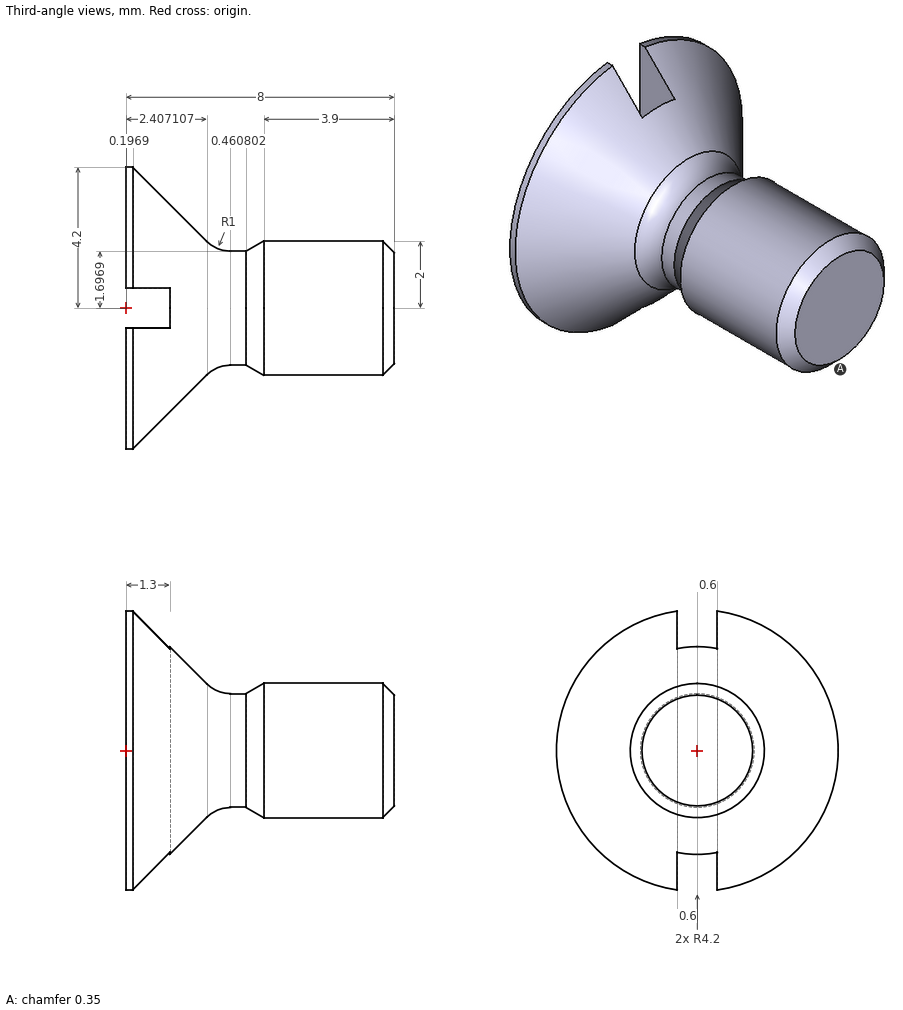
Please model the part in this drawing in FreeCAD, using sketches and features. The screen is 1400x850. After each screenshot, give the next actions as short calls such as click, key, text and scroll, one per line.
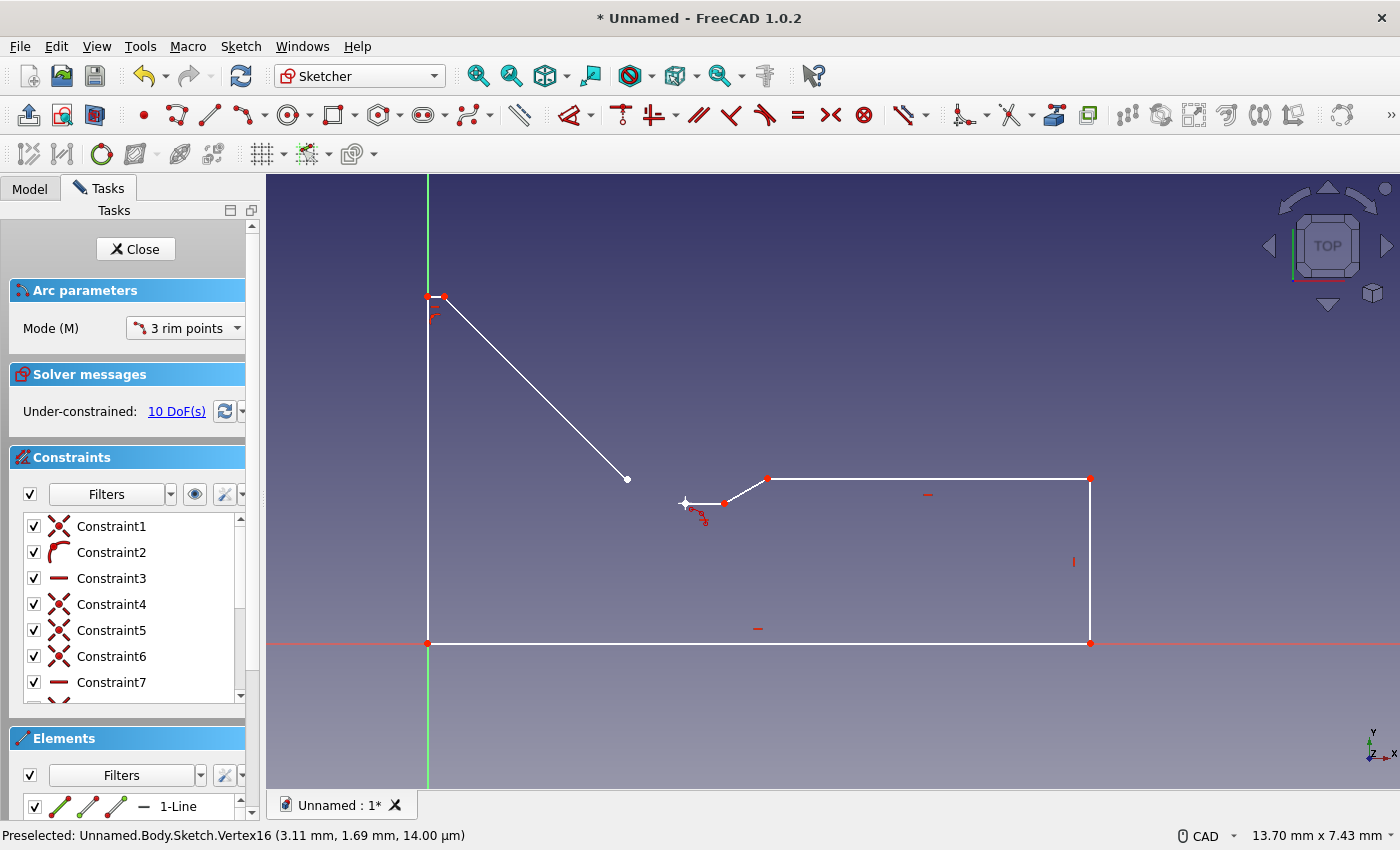
click(685, 504)
click(627, 480)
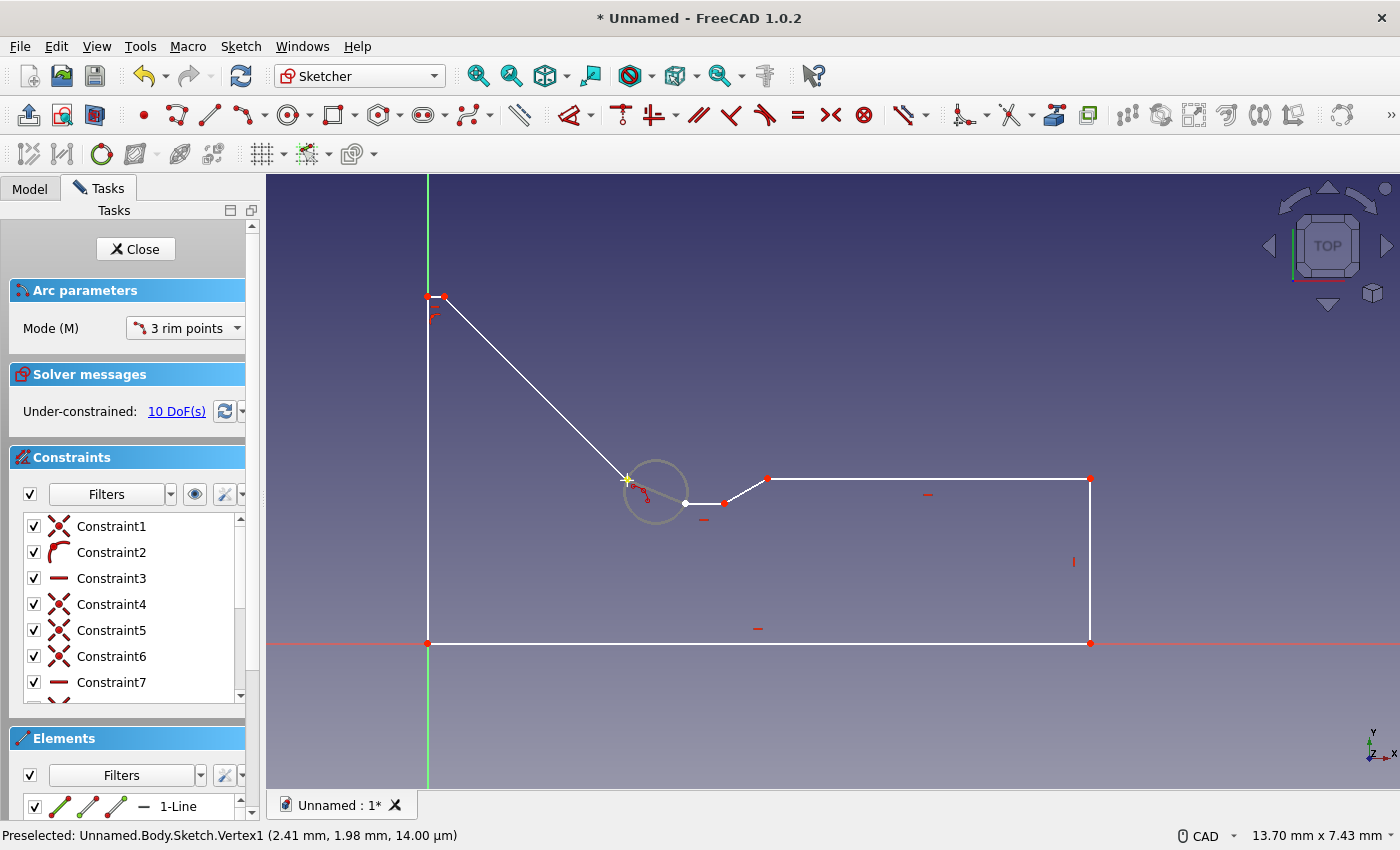
scroll(654, 497, up, 5)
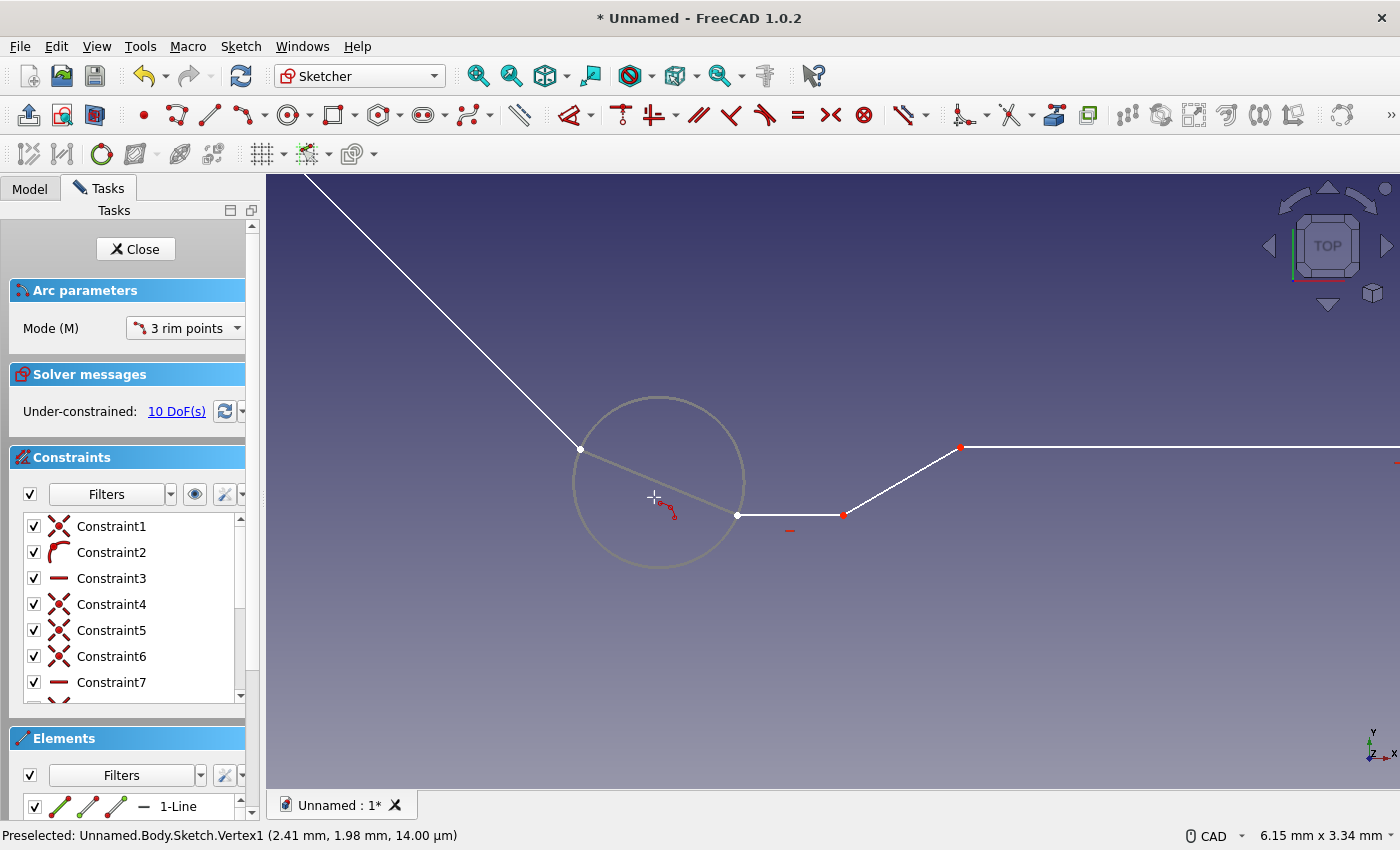
click(653, 496)
key(Escape)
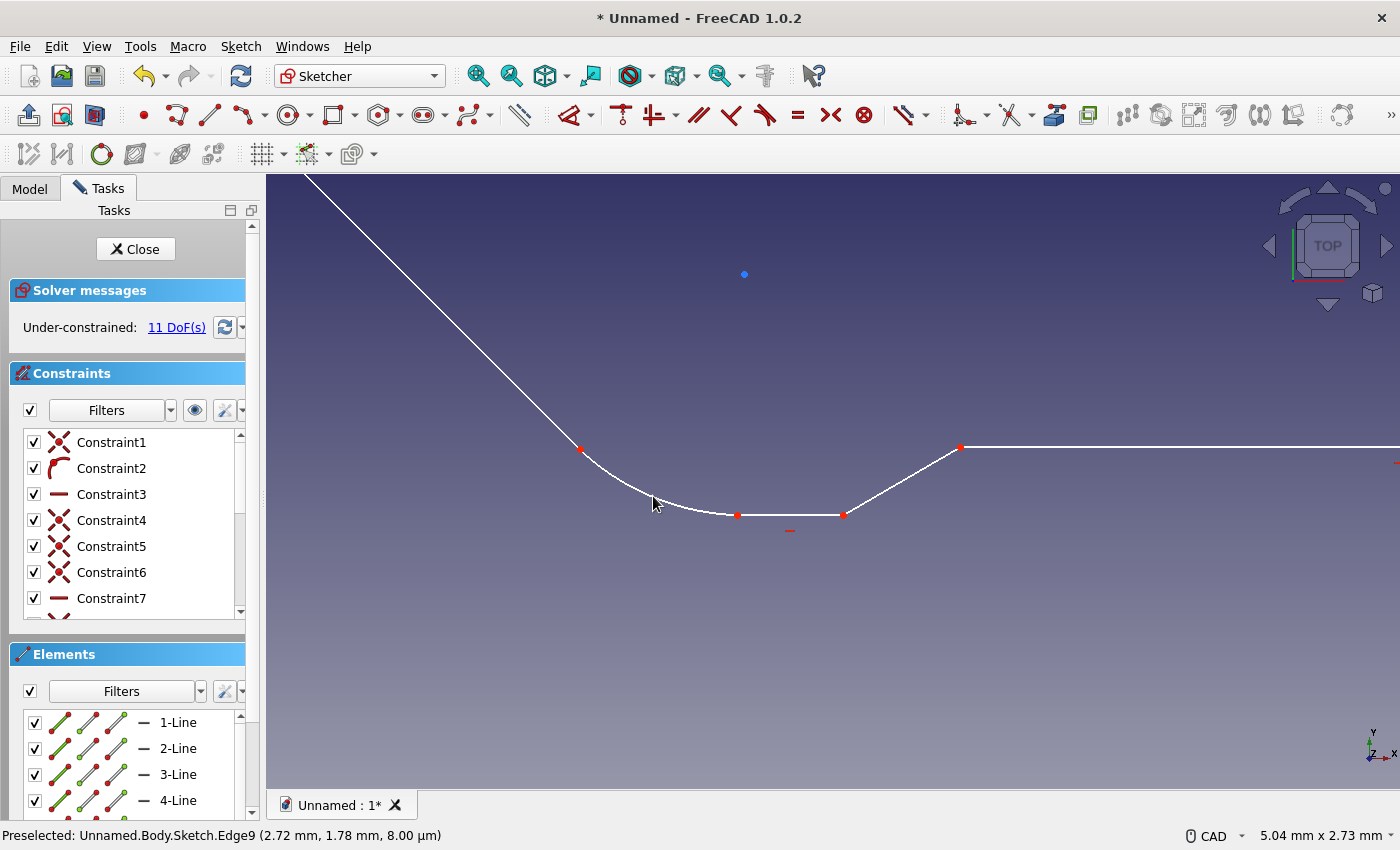
click(431, 301)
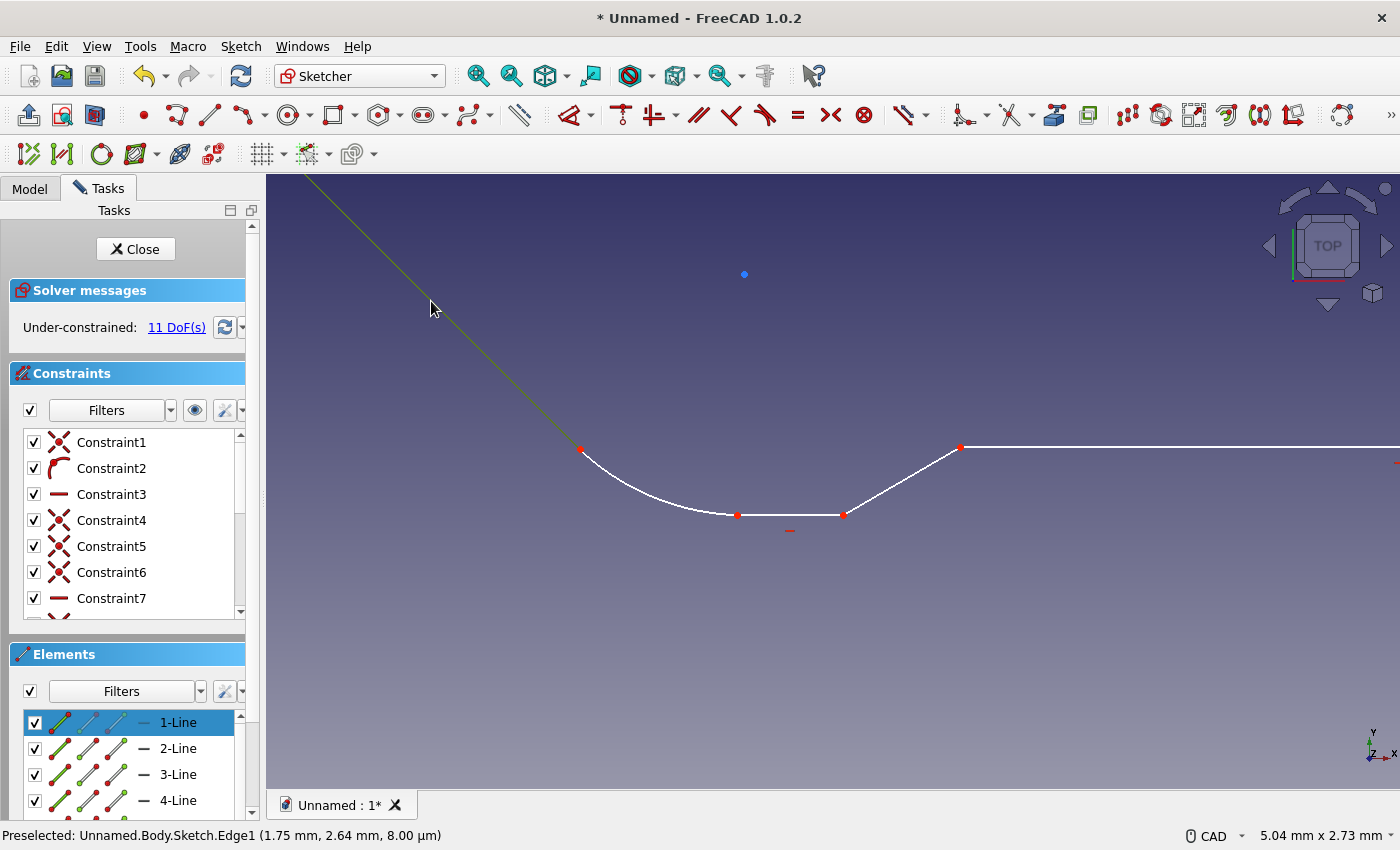
click(622, 481)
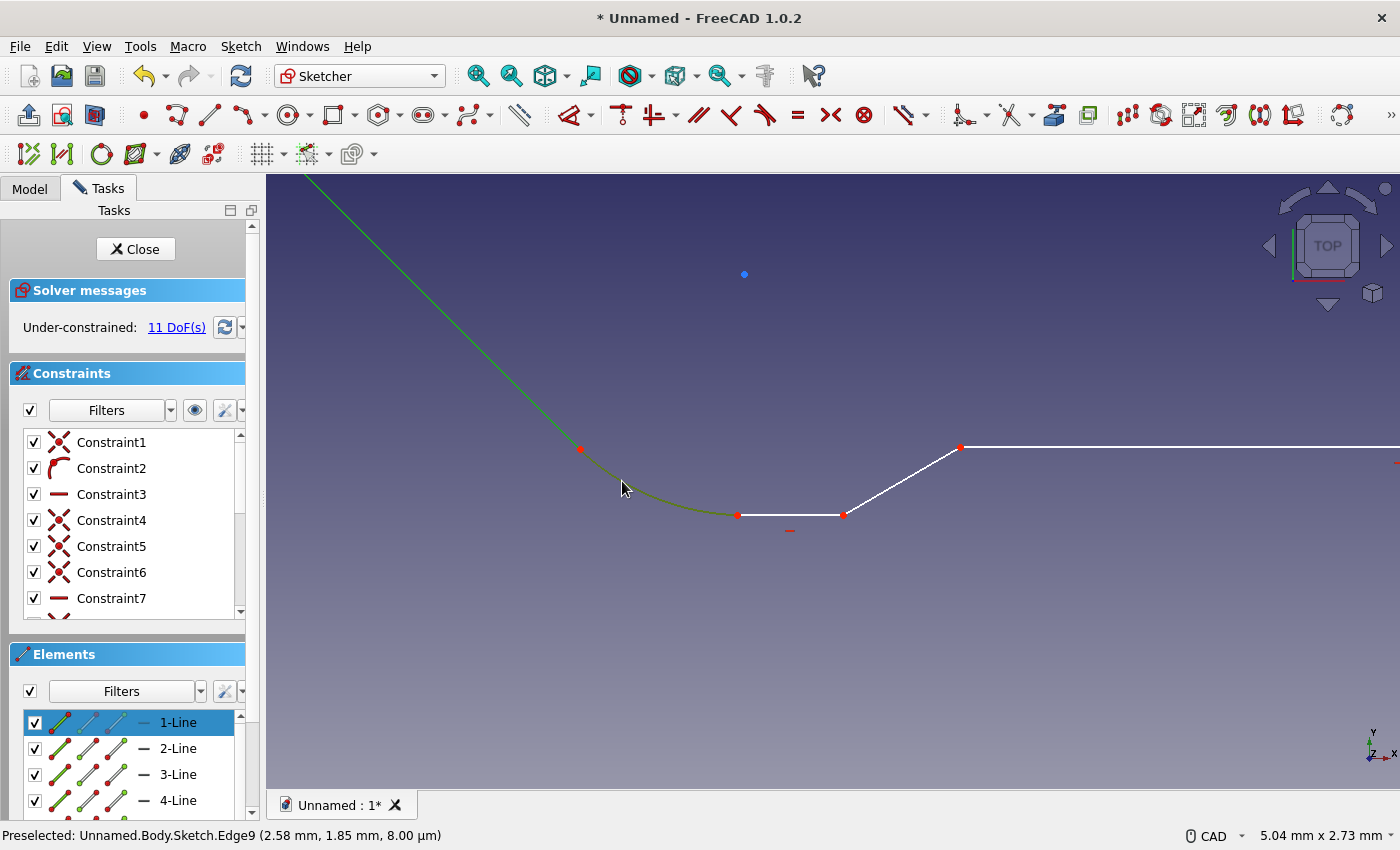
key(t)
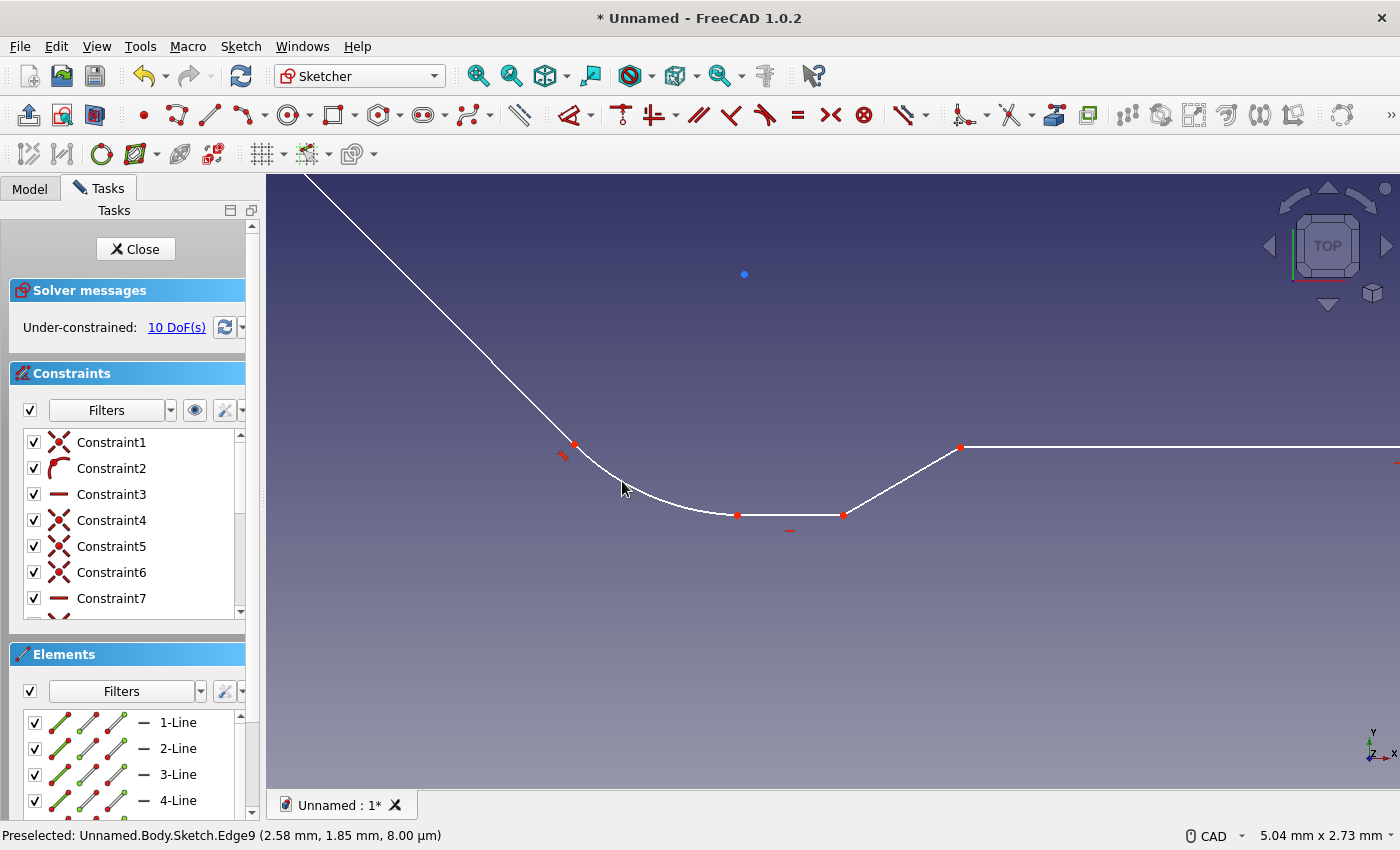
click(812, 515)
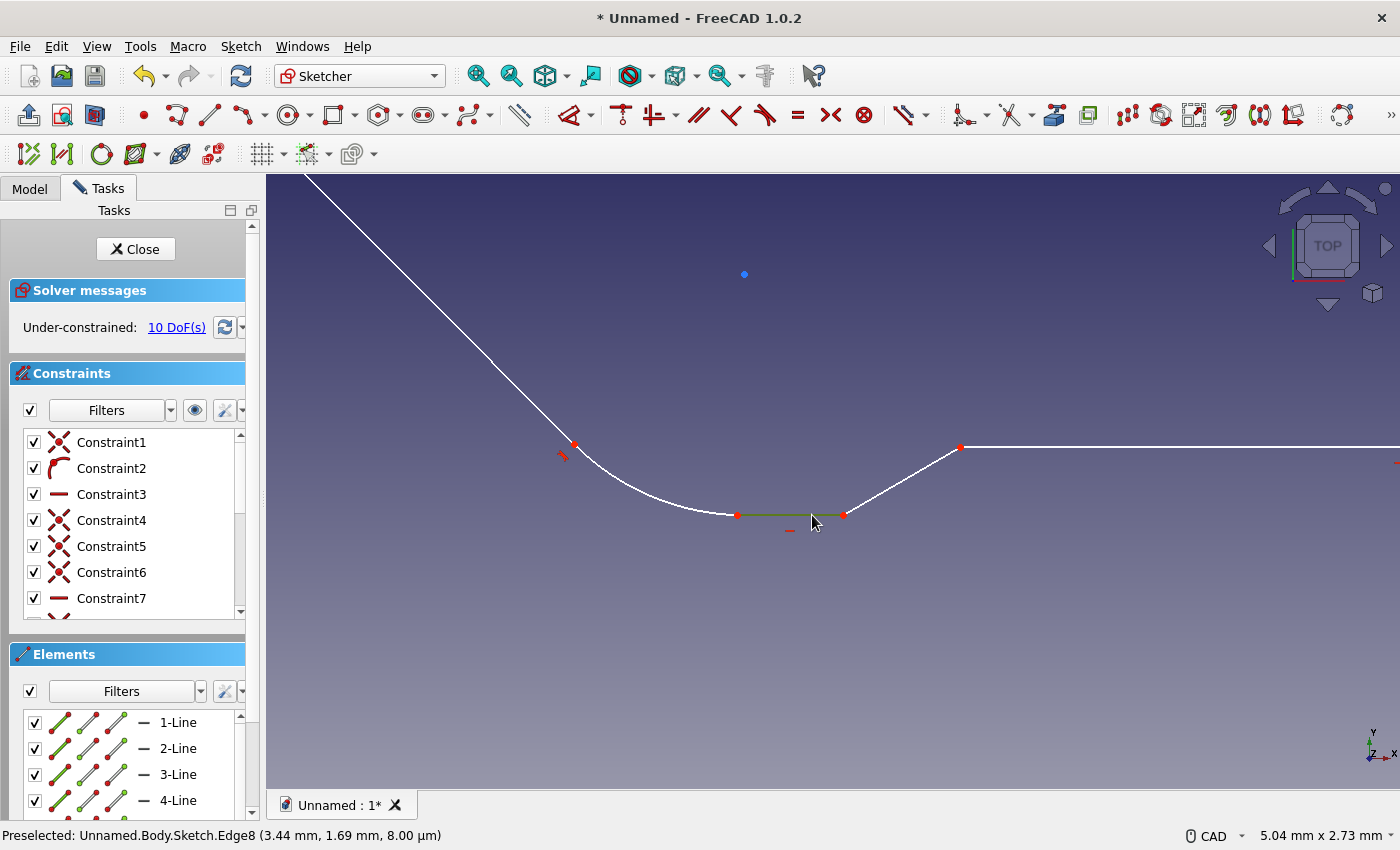
click(617, 479)